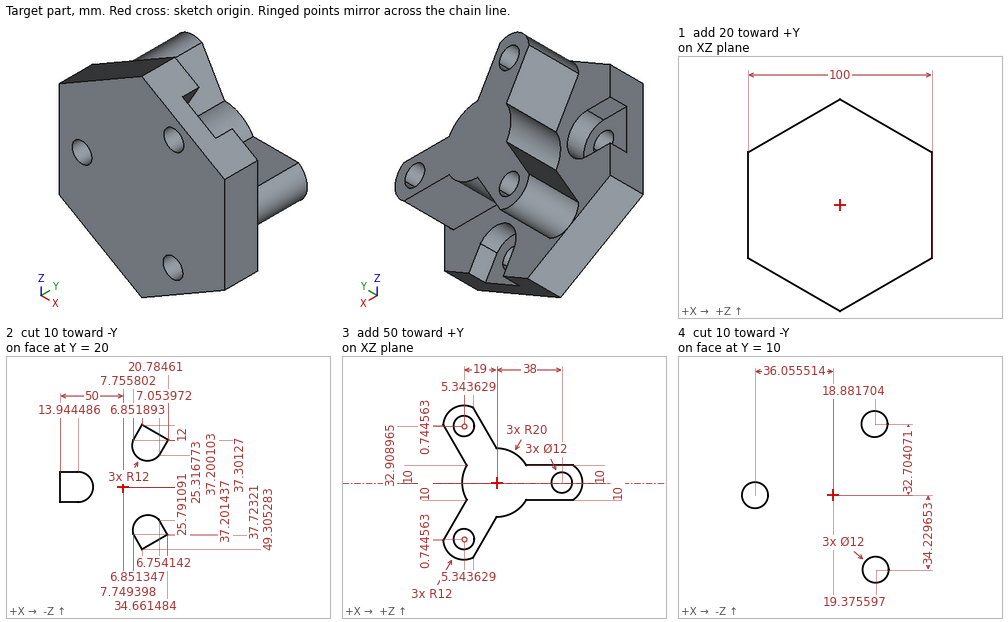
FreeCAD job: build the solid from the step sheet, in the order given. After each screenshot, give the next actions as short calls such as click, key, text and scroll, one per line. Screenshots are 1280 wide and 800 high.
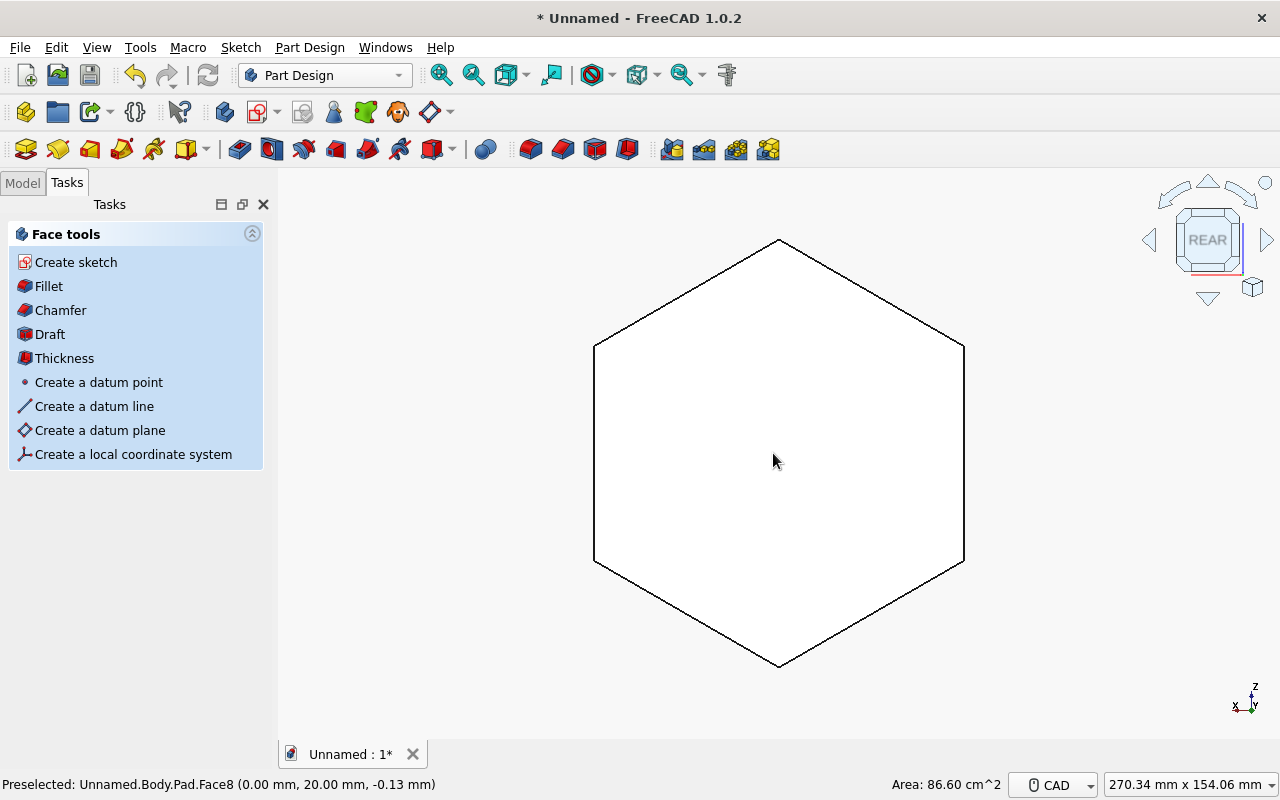
click(258, 112)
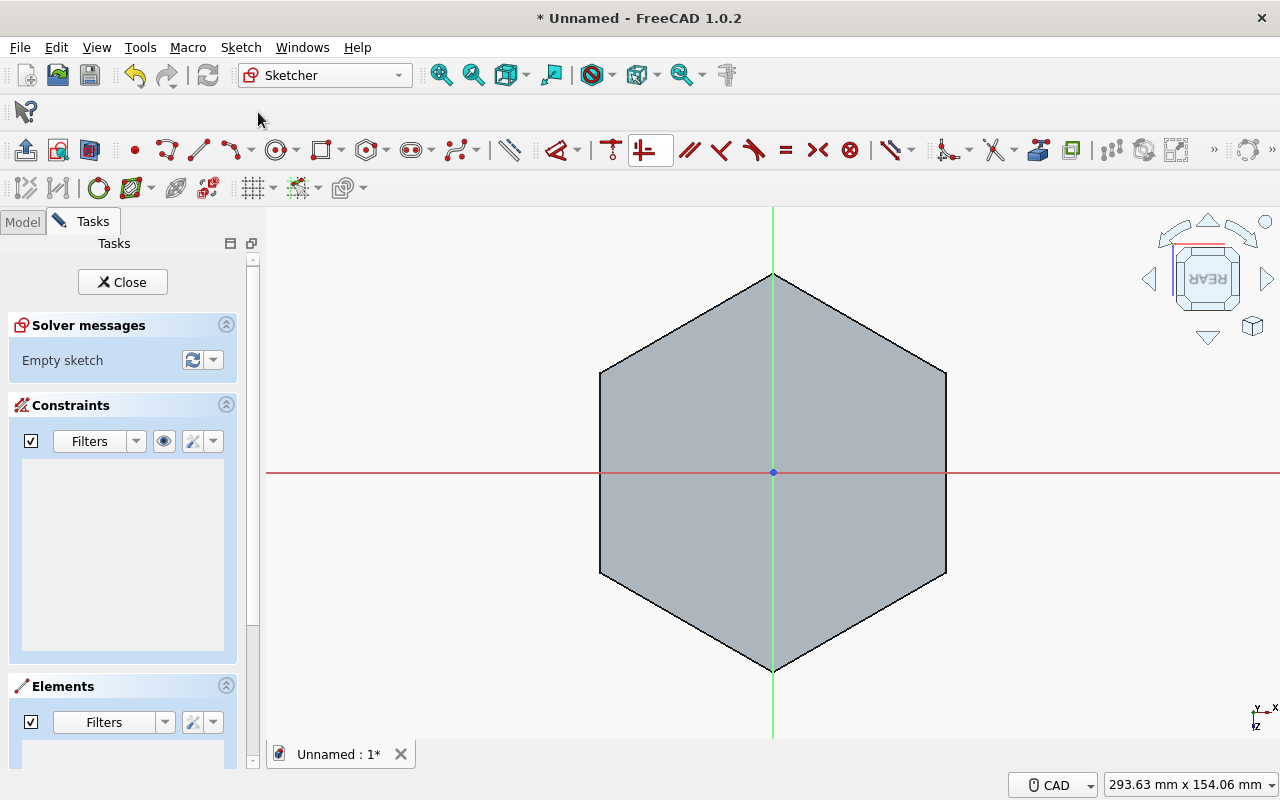
click(168, 150)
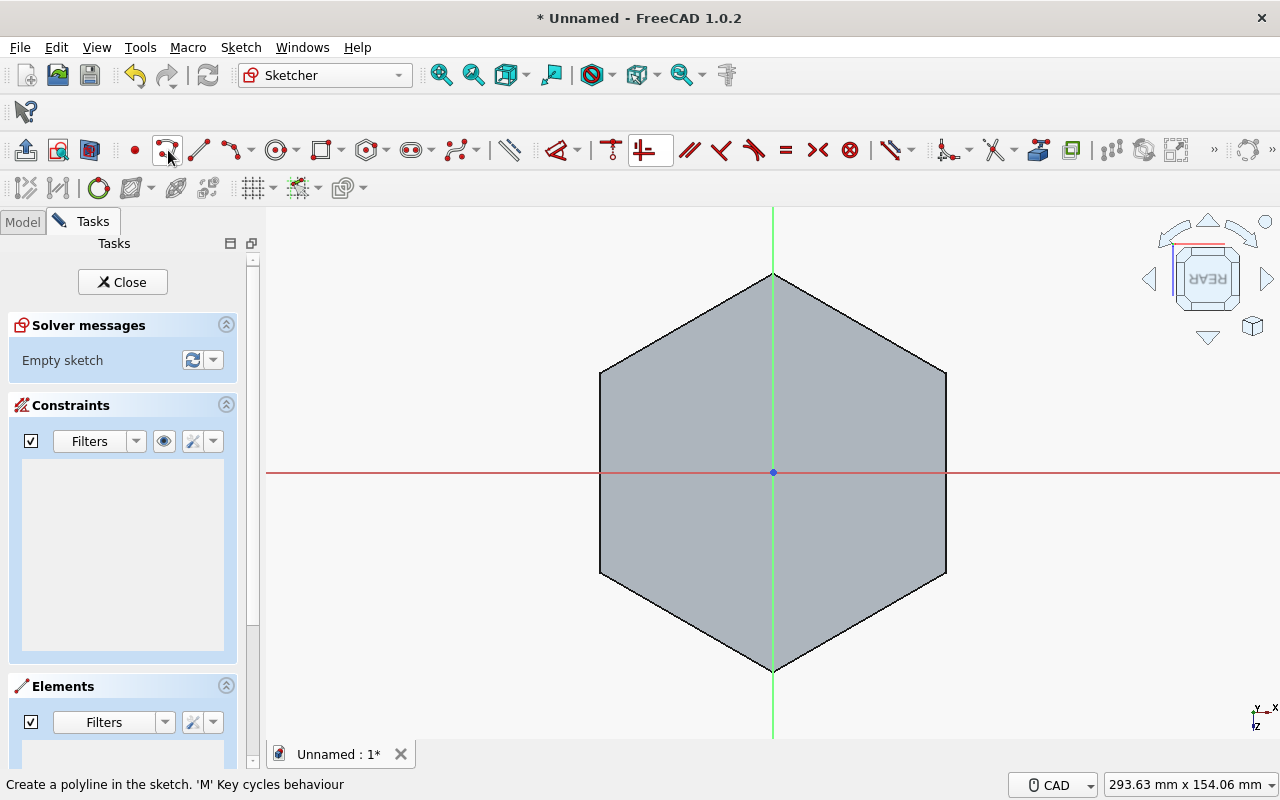
click(648, 432)
click(600, 432)
click(600, 514)
click(648, 514)
right_click(648, 514)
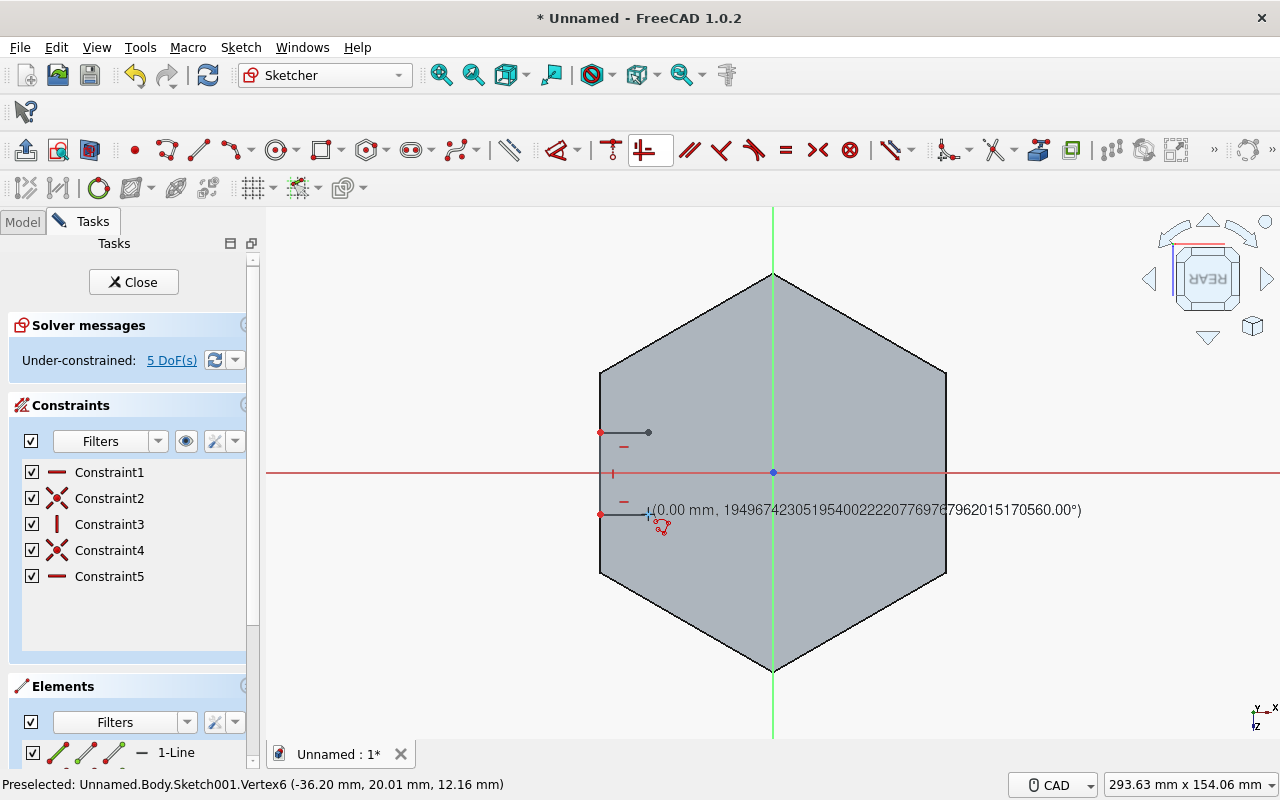
click(232, 150)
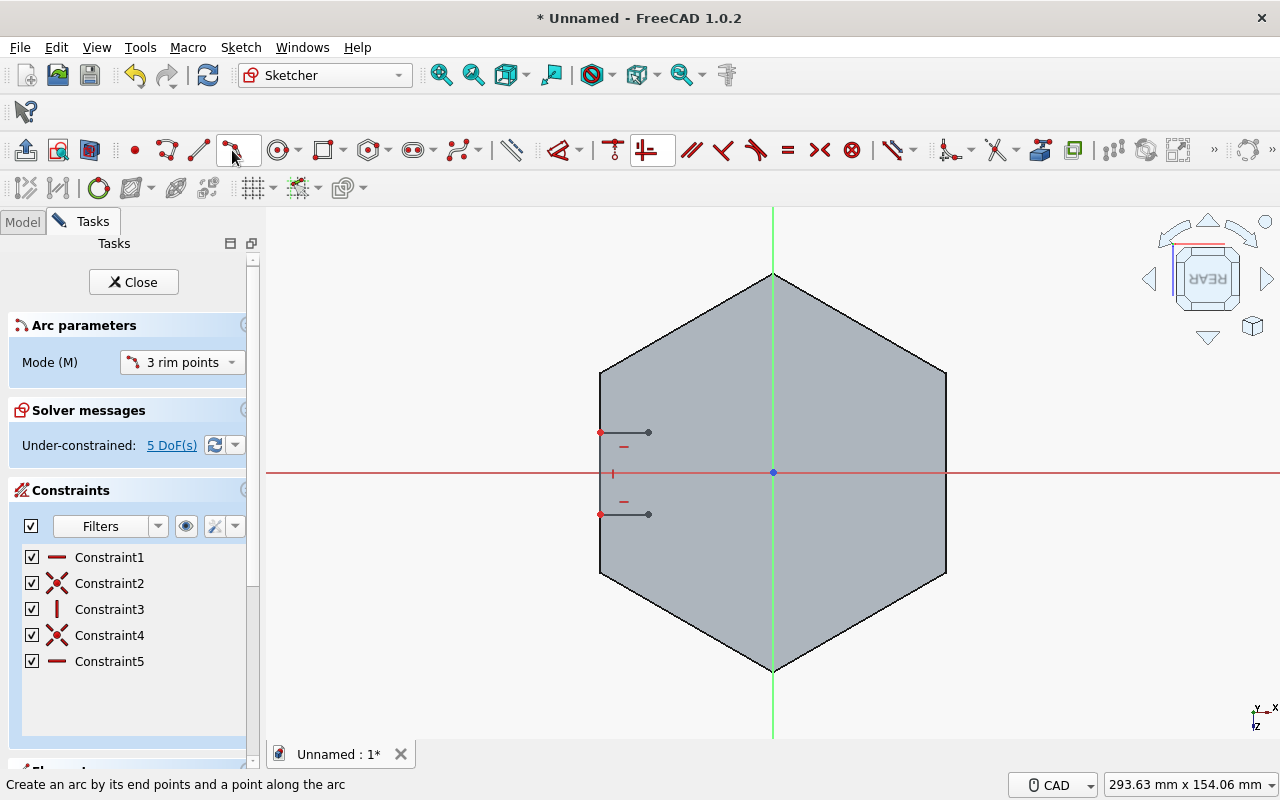
click(648, 515)
click(648, 433)
click(682, 497)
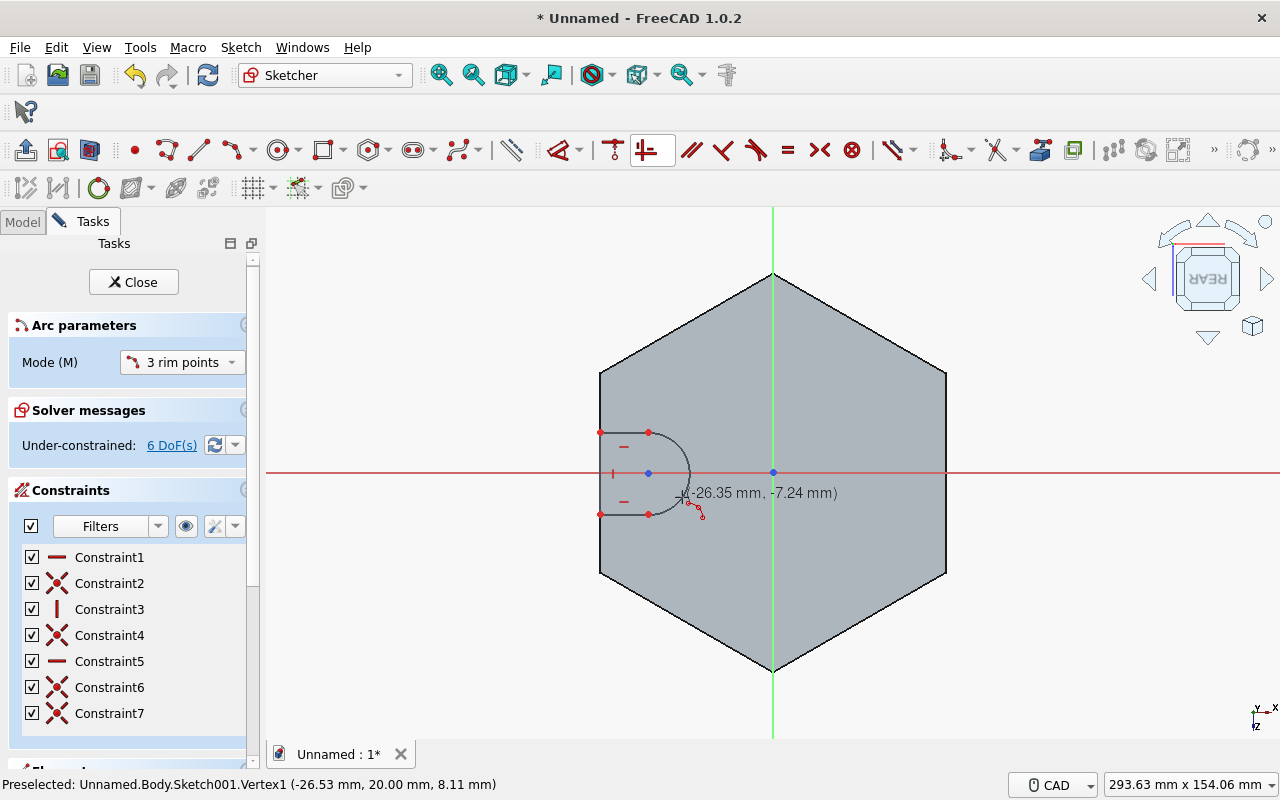
click(168, 150)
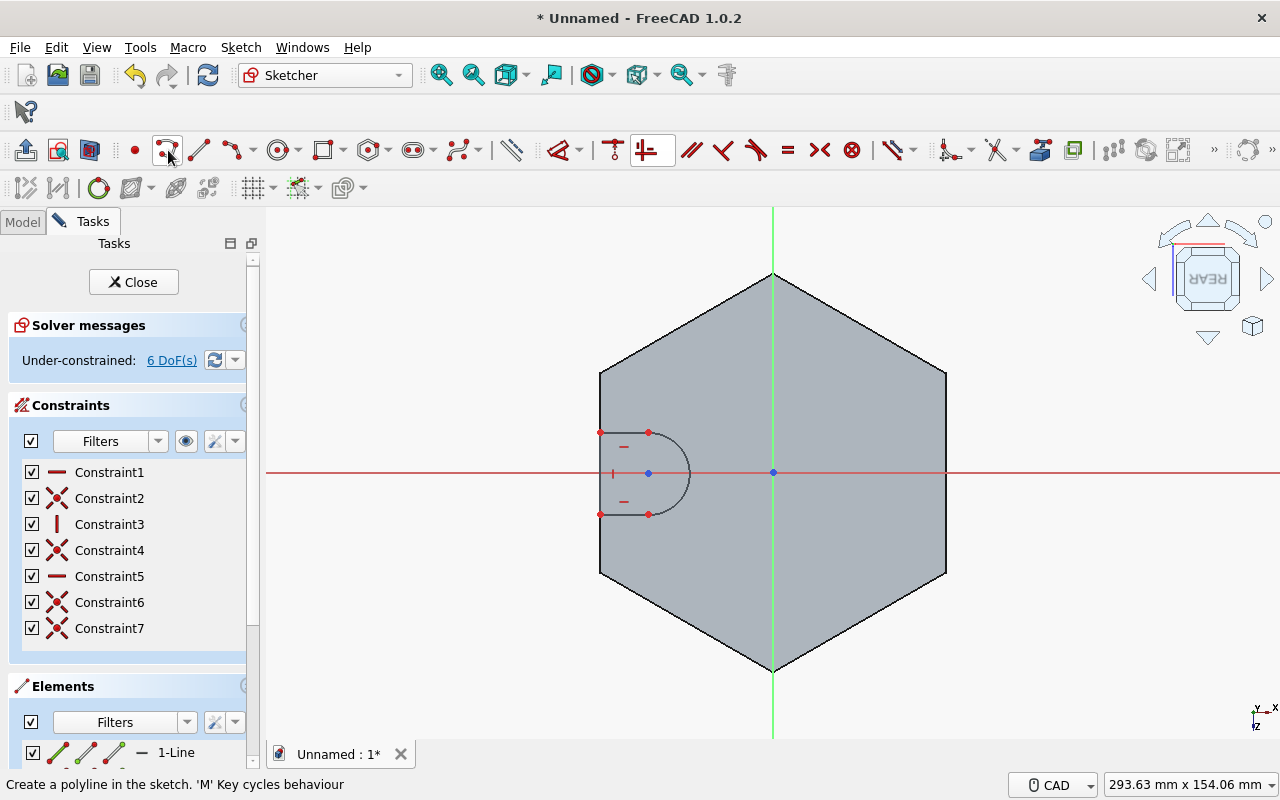
click(871, 386)
click(895, 344)
click(823, 303)
click(800, 345)
right_click(800, 345)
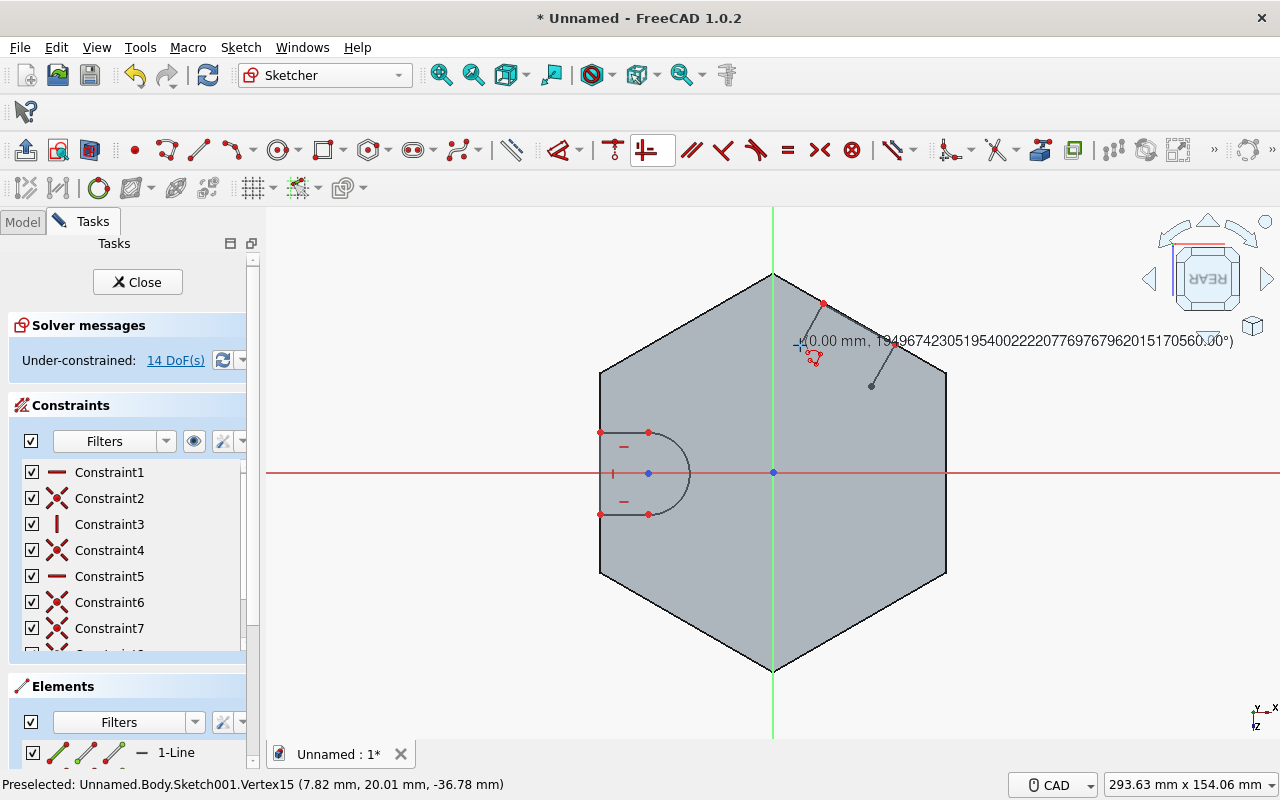
click(232, 150)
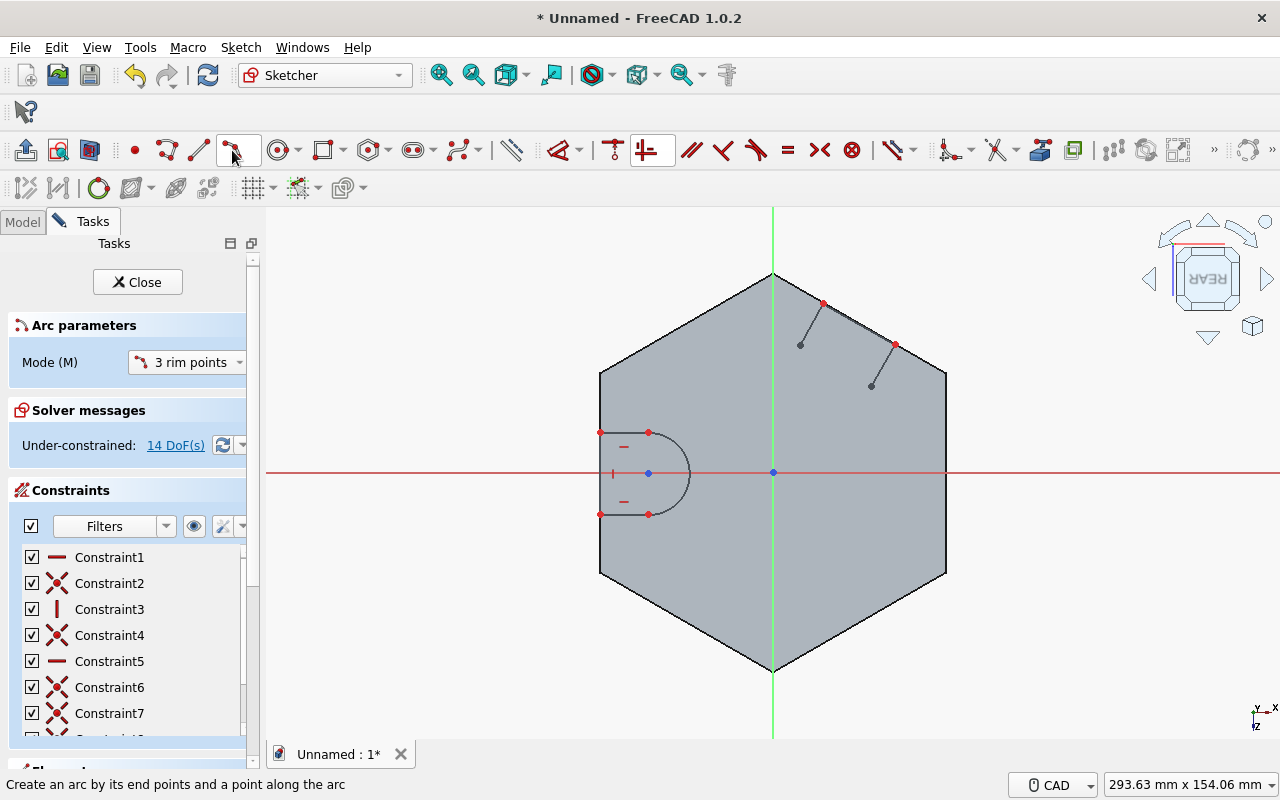
click(800, 346)
click(871, 387)
click(817, 396)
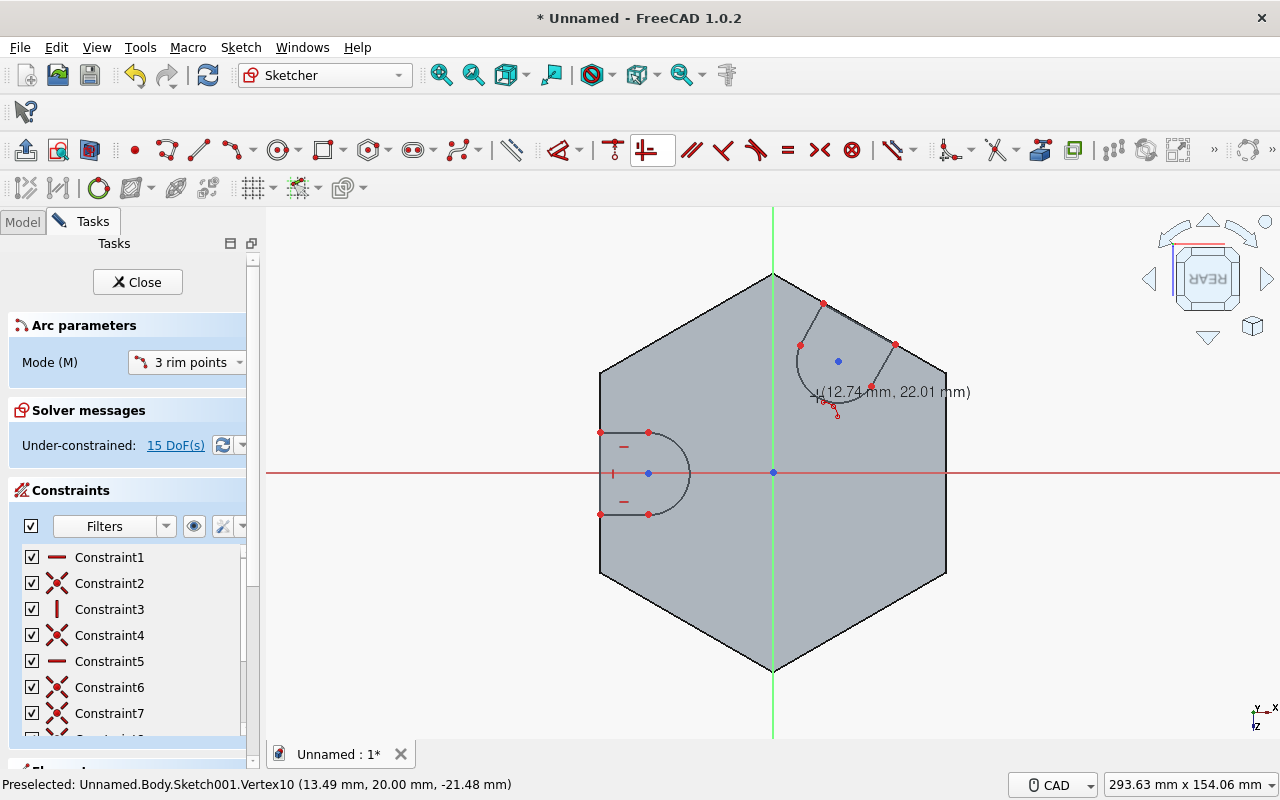
click(168, 150)